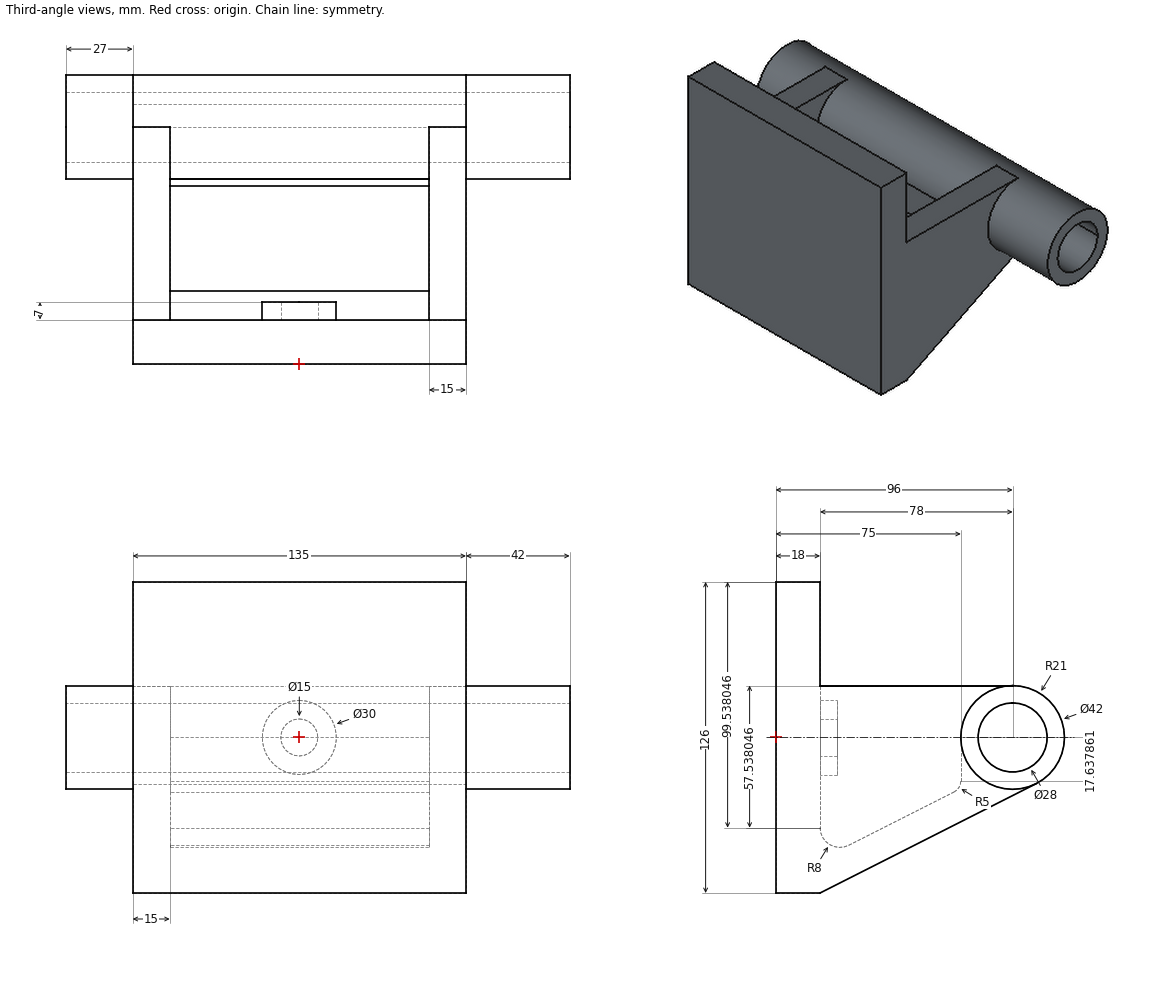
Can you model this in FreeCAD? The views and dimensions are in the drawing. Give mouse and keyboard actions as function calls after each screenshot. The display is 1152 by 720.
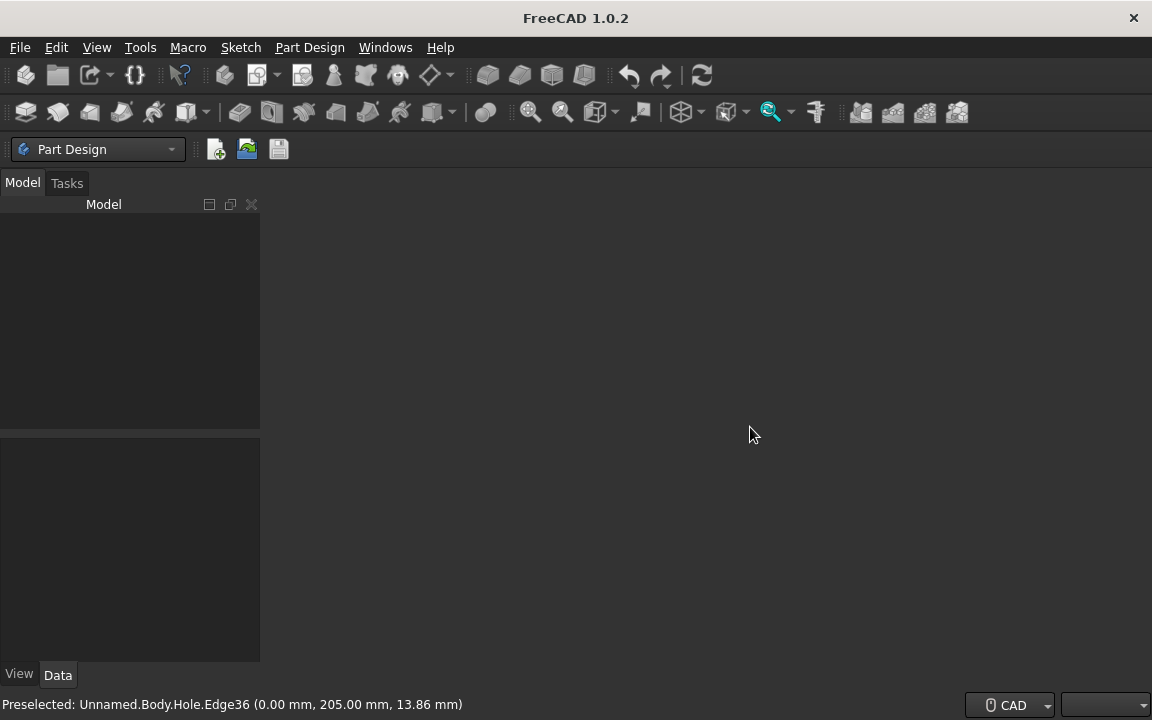
click(216, 150)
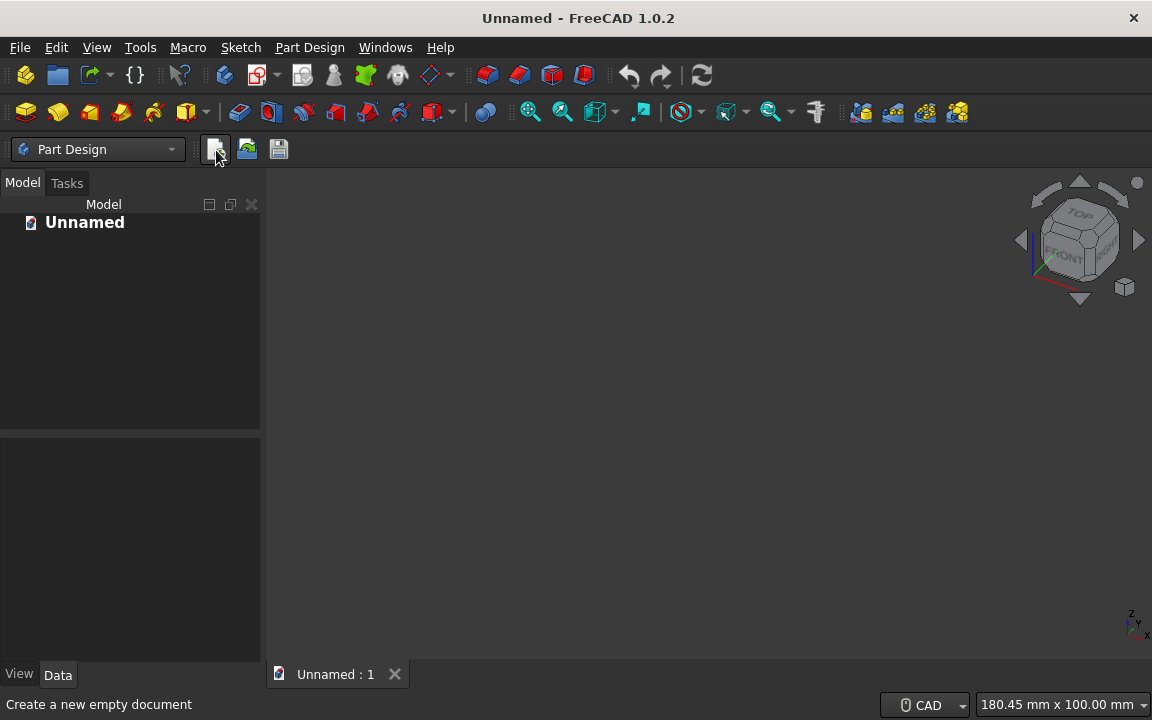
click(258, 76)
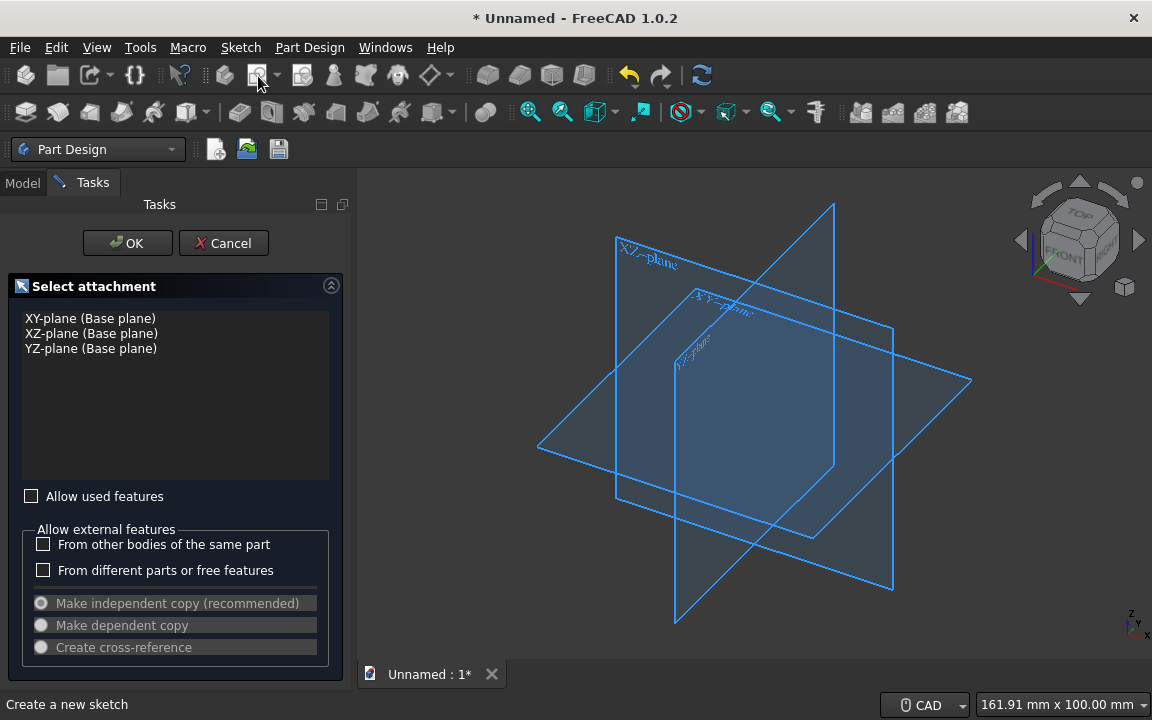
click(82, 348)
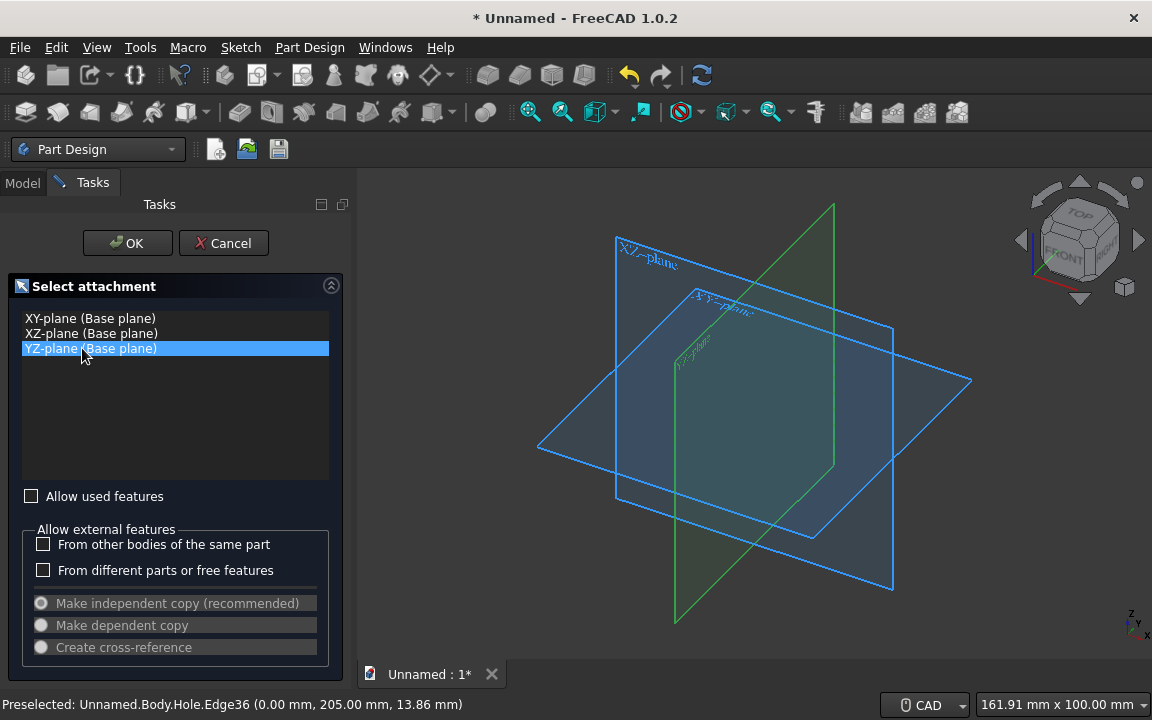
click(128, 243)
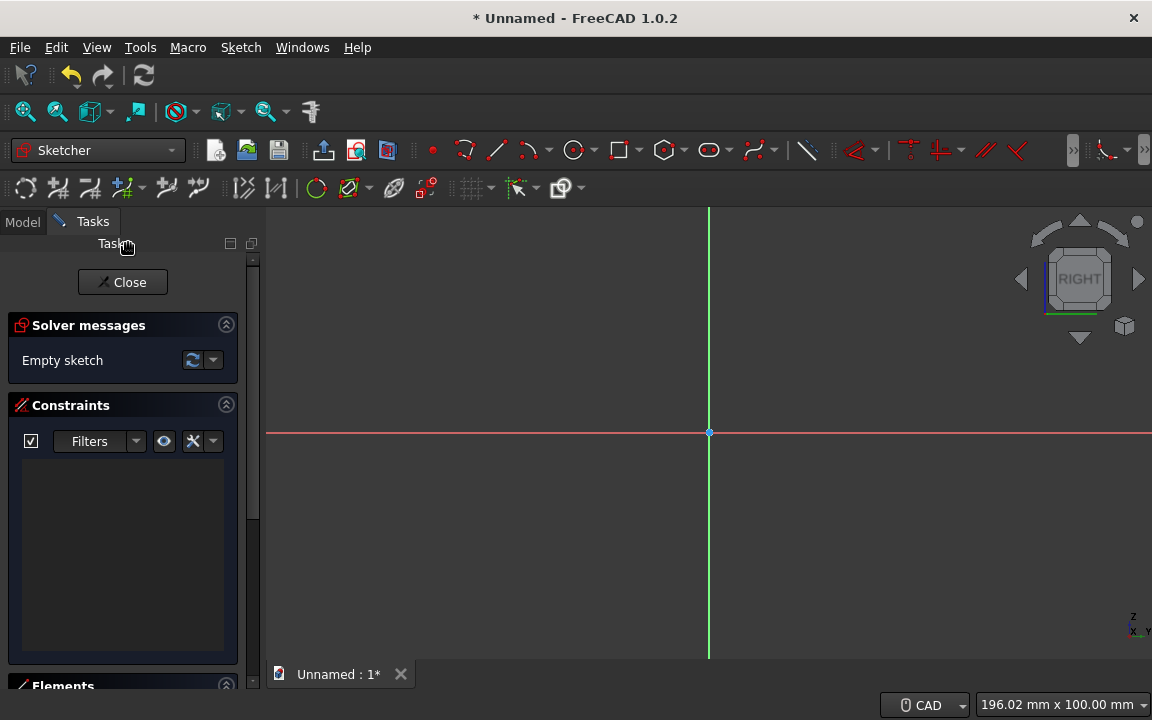
scroll(382, 433, down, 4)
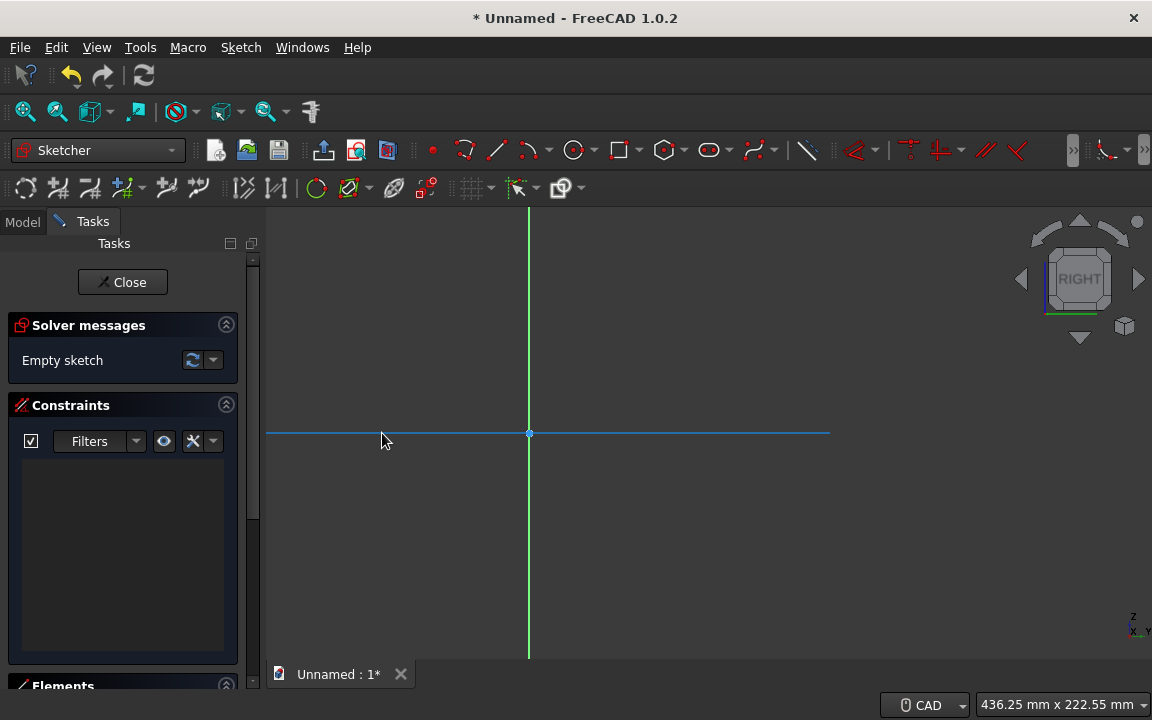
click(498, 150)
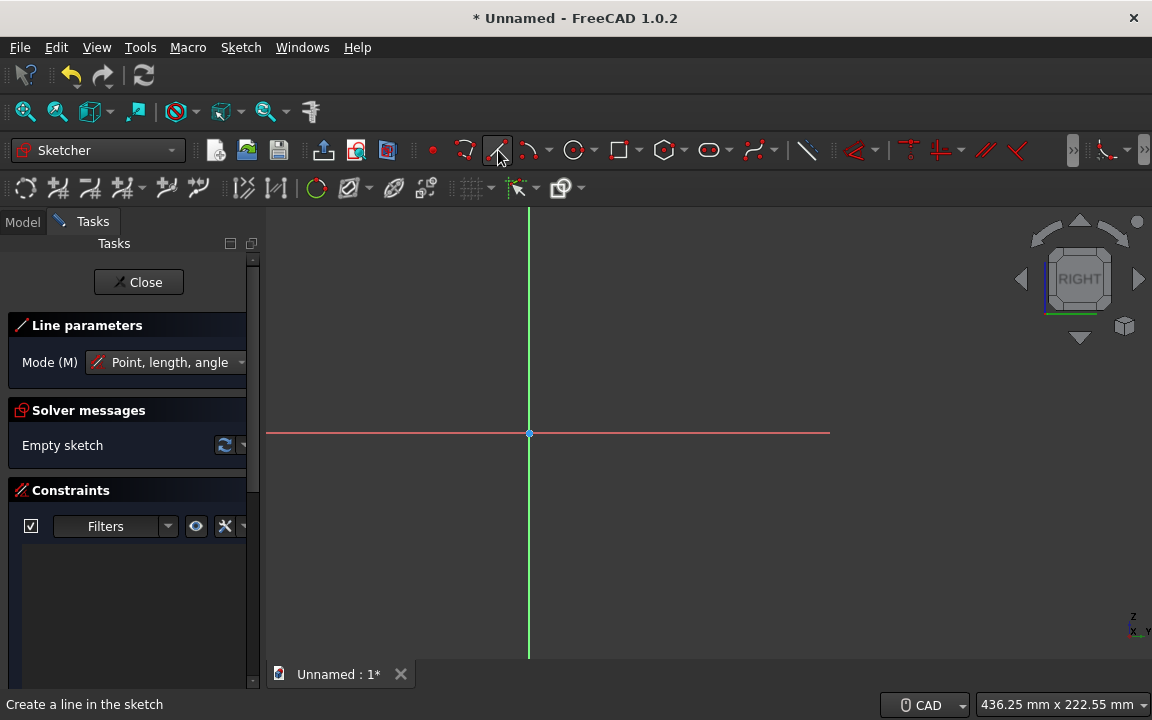
click(681, 433)
click(681, 469)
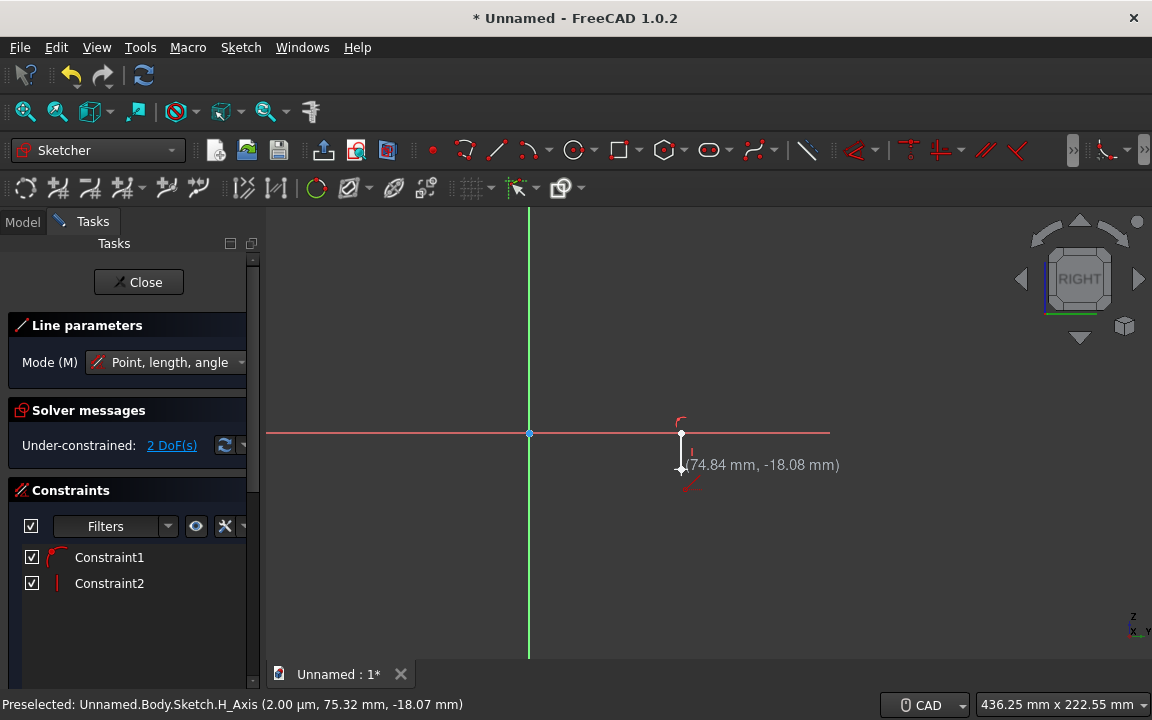
scroll(676, 478, up, 3)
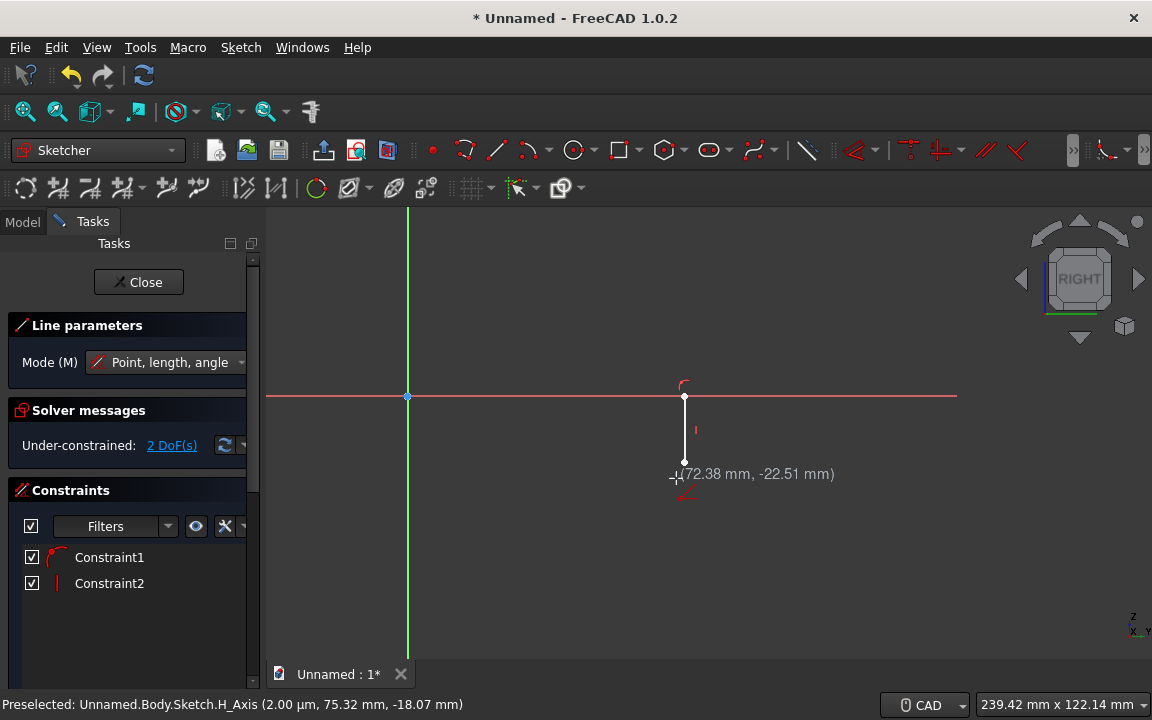
click(675, 478)
click(517, 558)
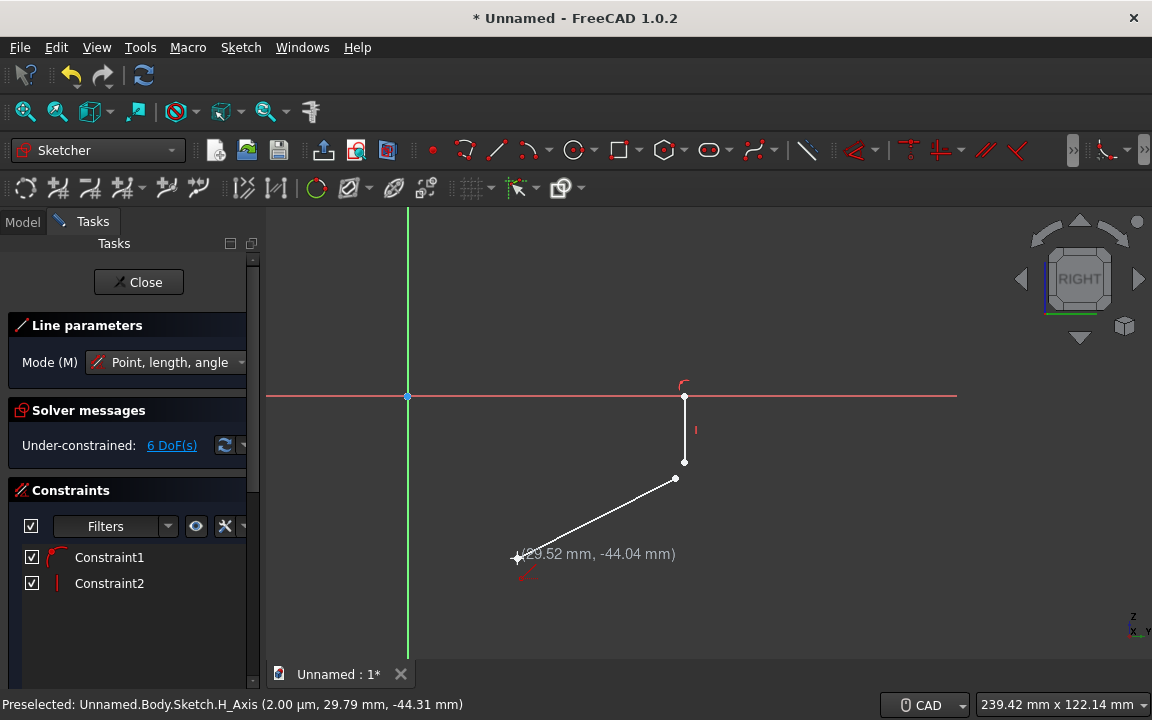
click(466, 150)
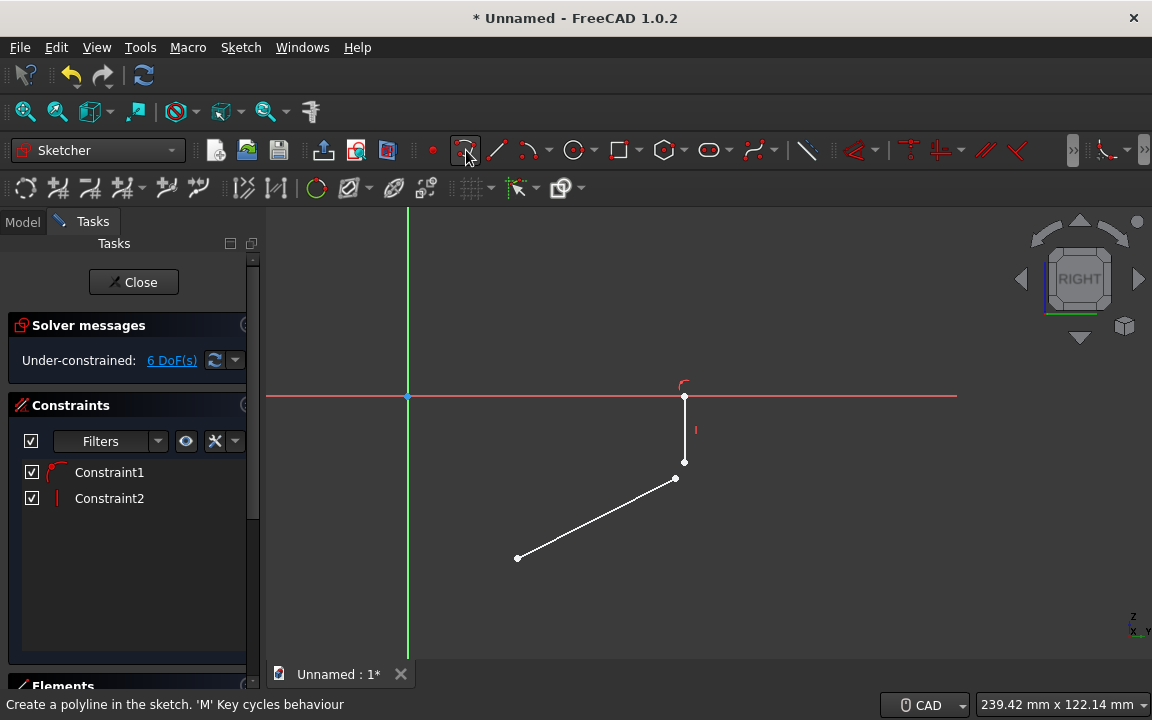
click(474, 531)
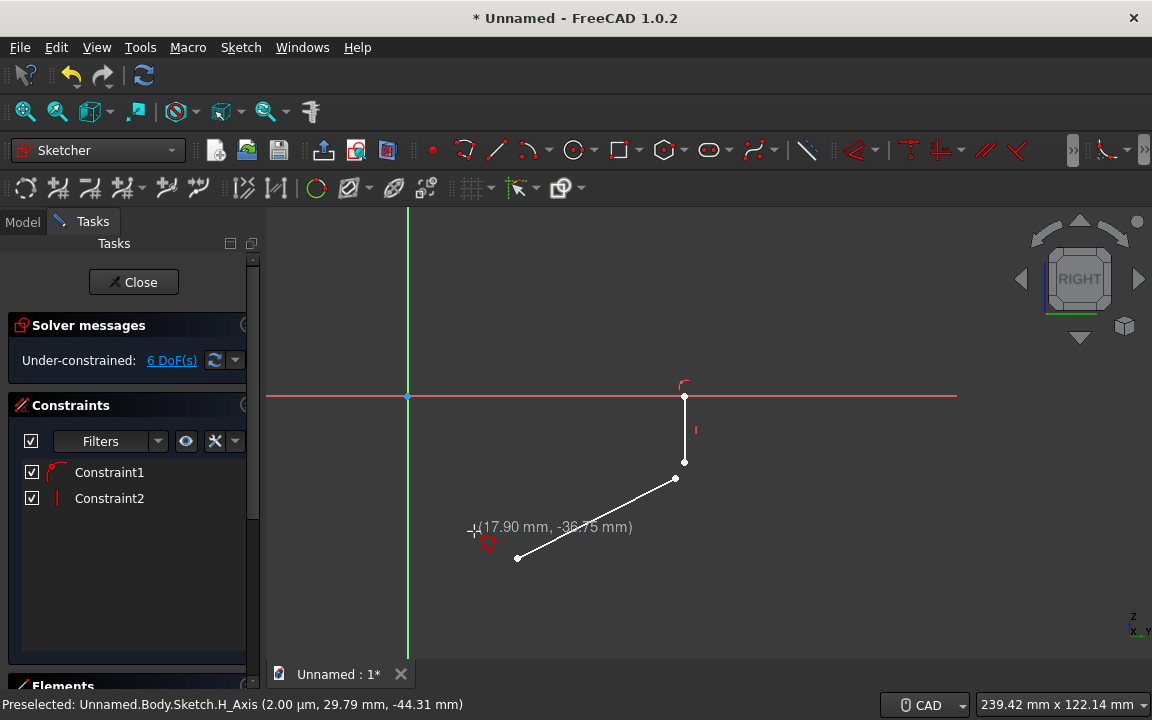
scroll(676, 478, down, 3)